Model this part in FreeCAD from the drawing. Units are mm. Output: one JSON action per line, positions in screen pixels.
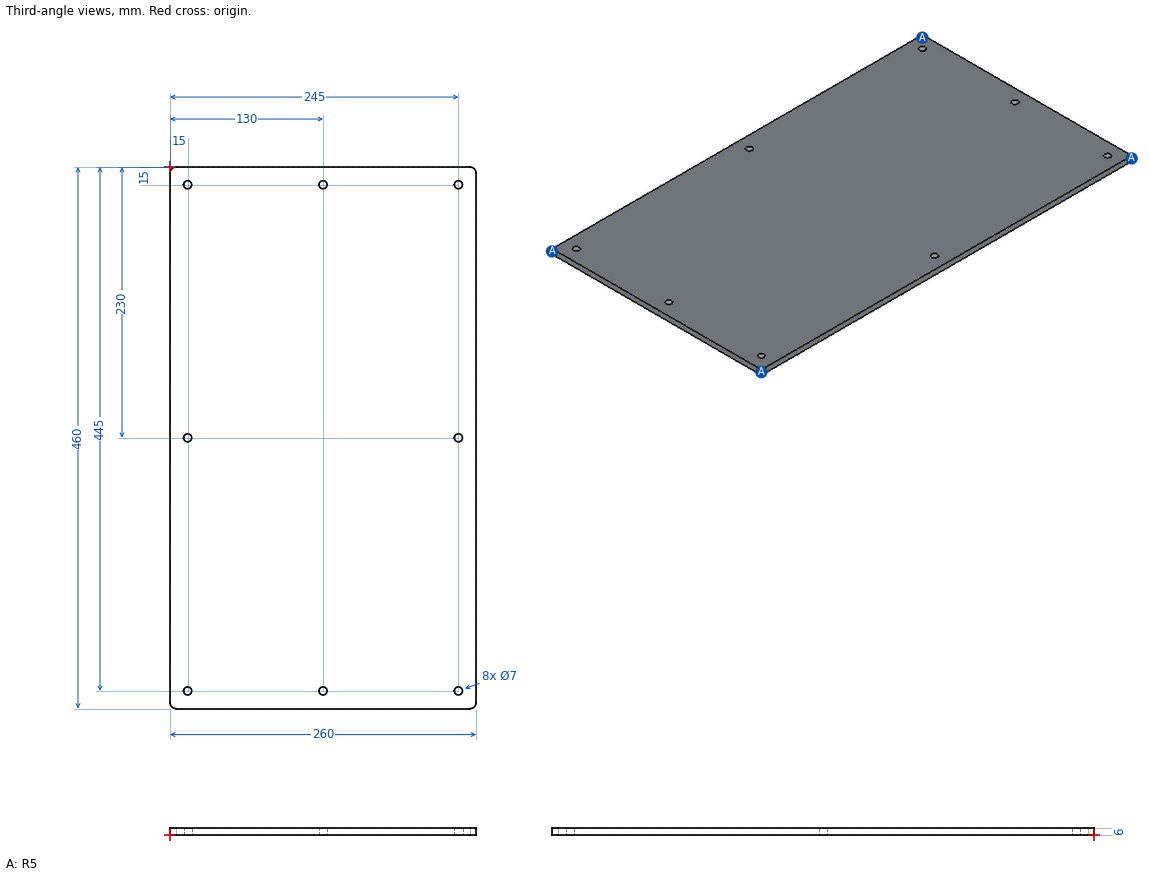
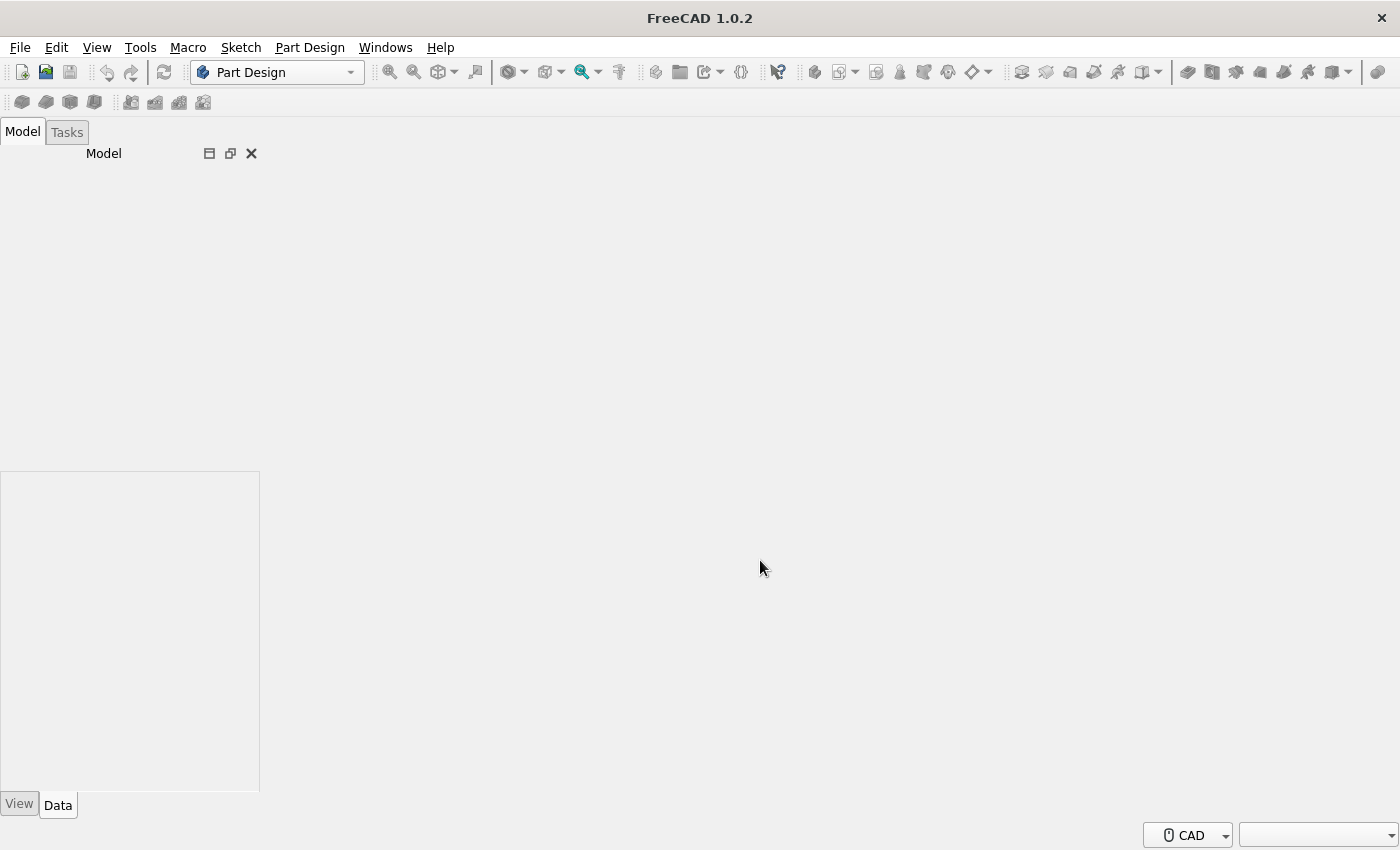
{"action": "key", "text": "ctrl+n"}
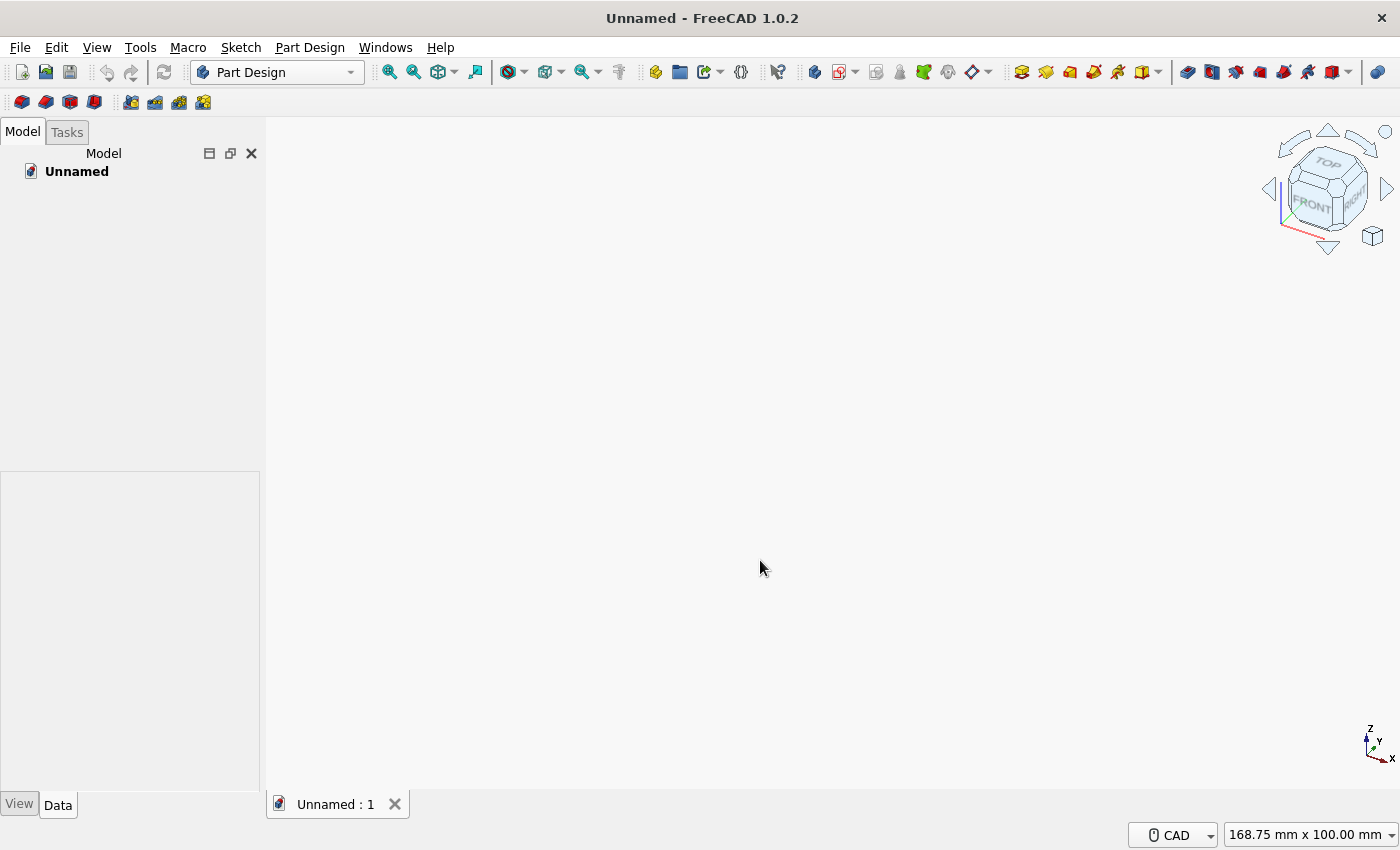
{"action": "left_click", "coordinate": [840, 72]}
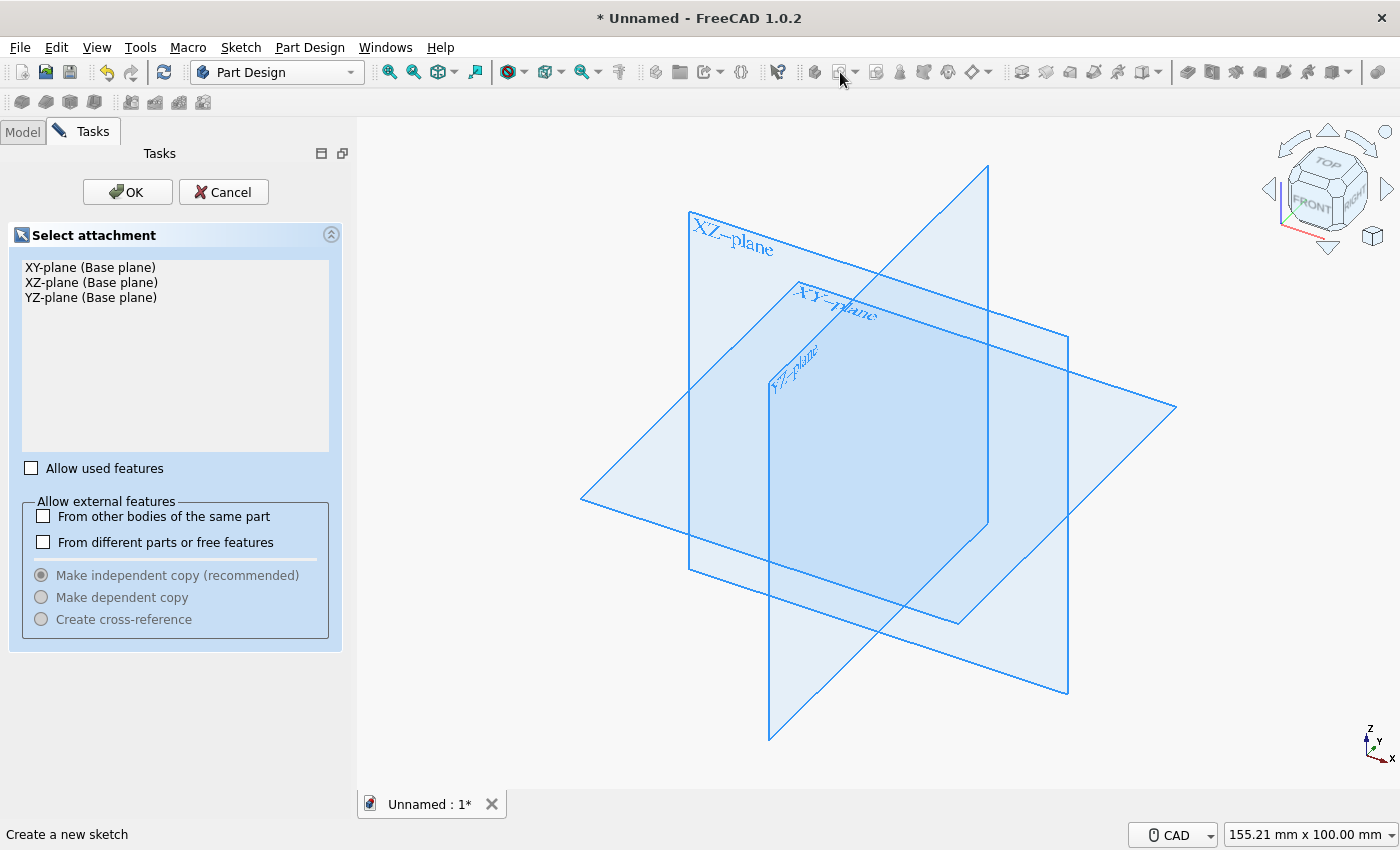
{"action": "left_click", "coordinate": [82, 268]}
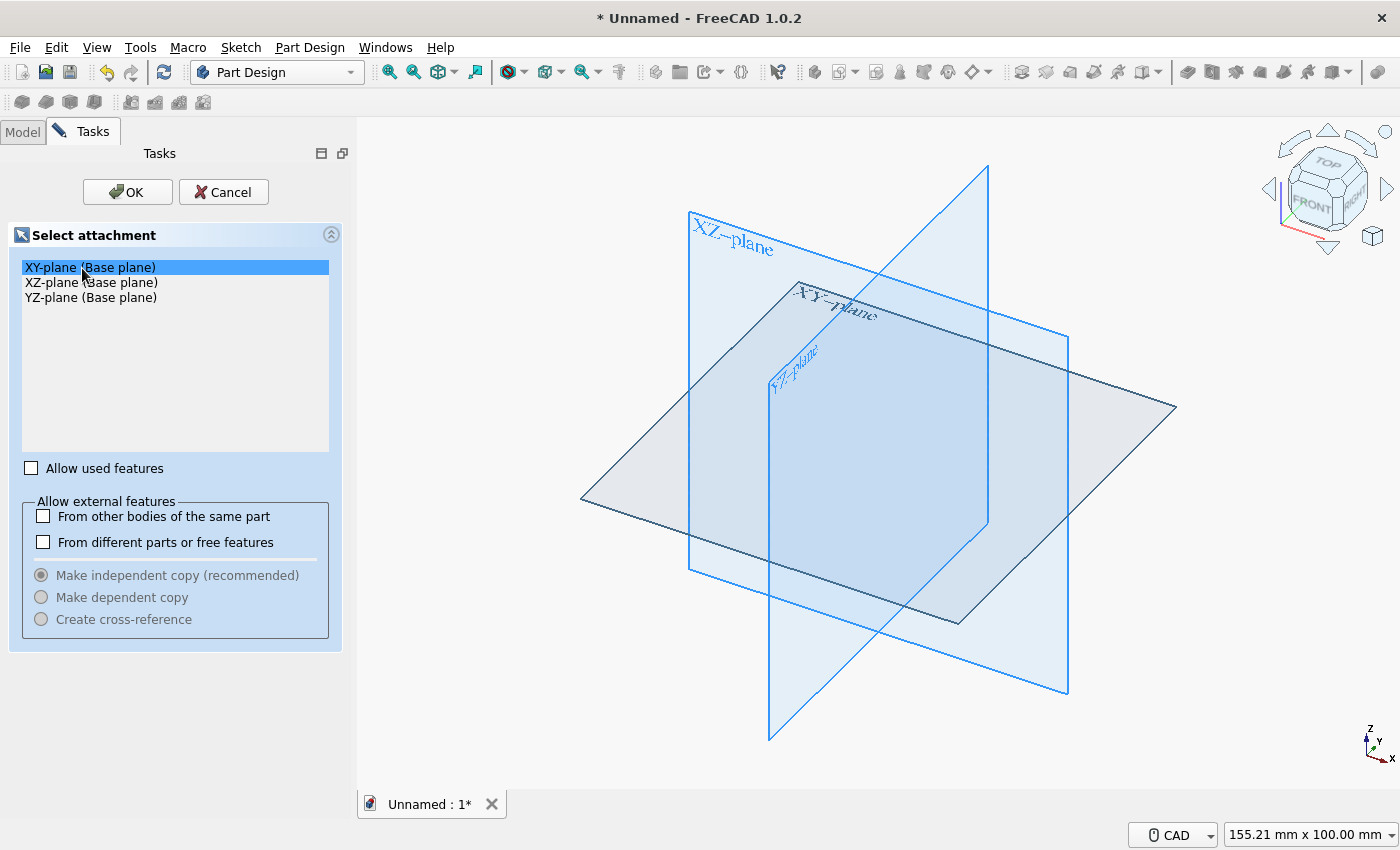
{"action": "left_click", "coordinate": [128, 192]}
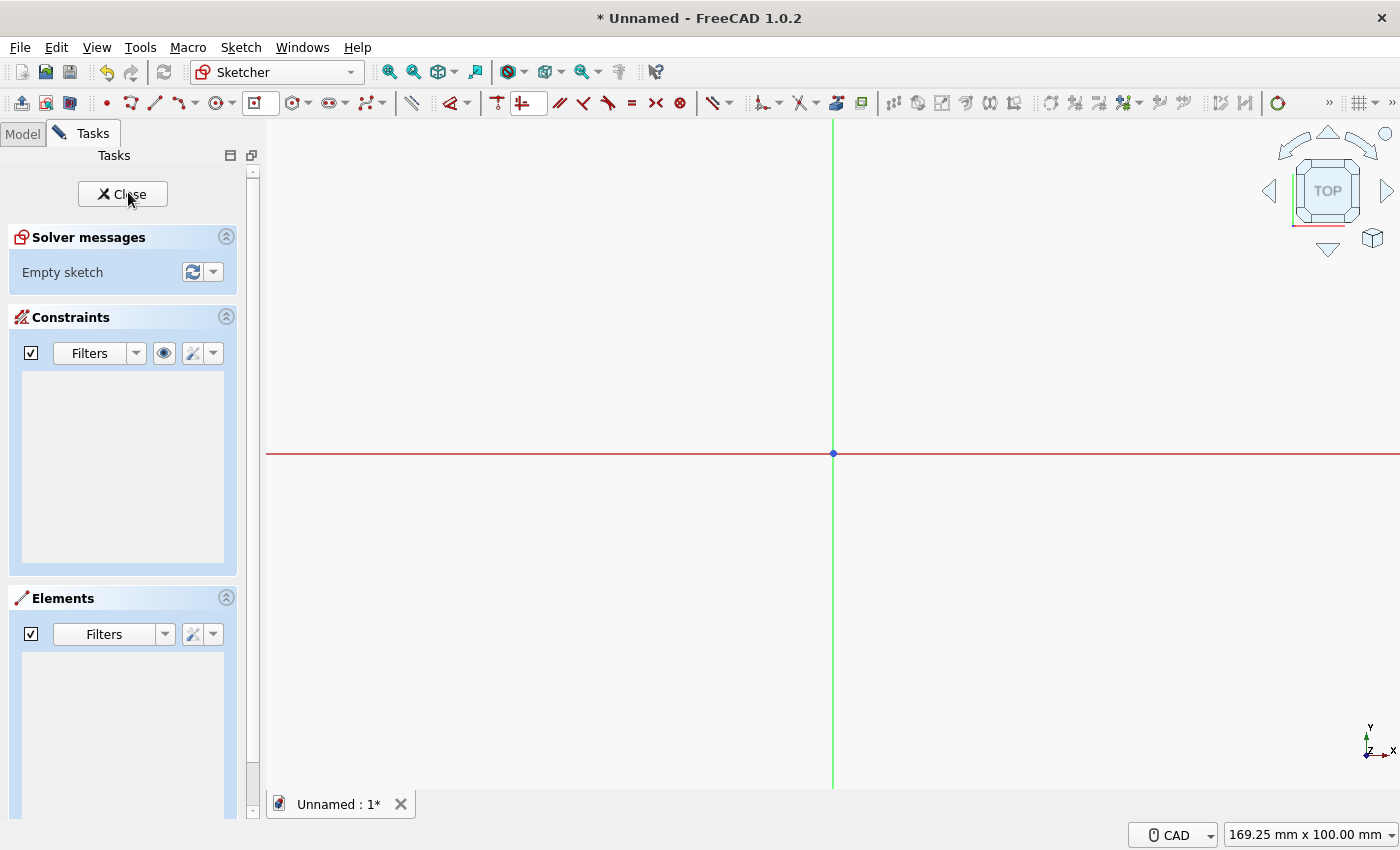
{"action": "scroll", "coordinate": [617, 213], "scroll_direction": "down", "scroll_amount": 10}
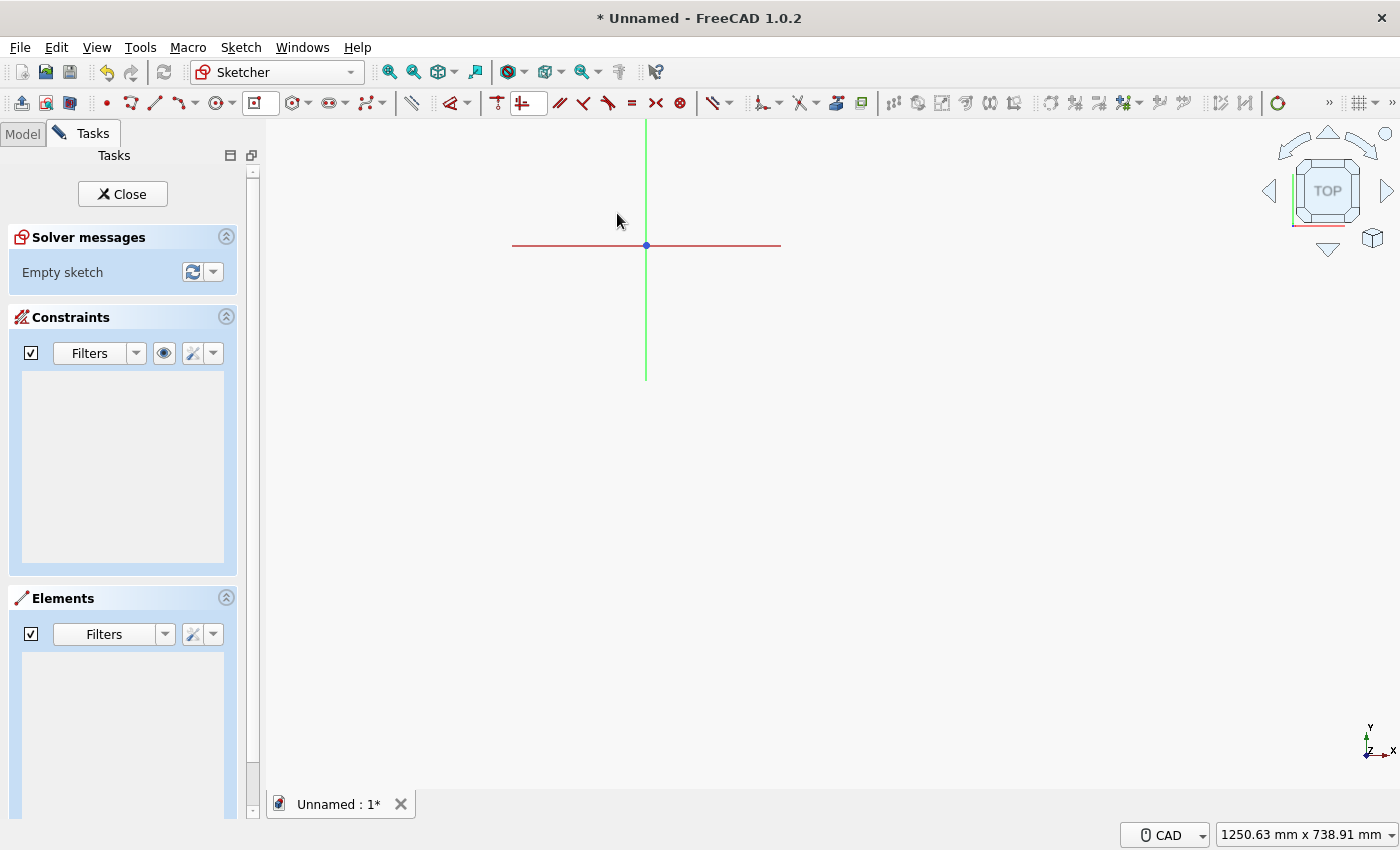
{"action": "key", "text": "g r"}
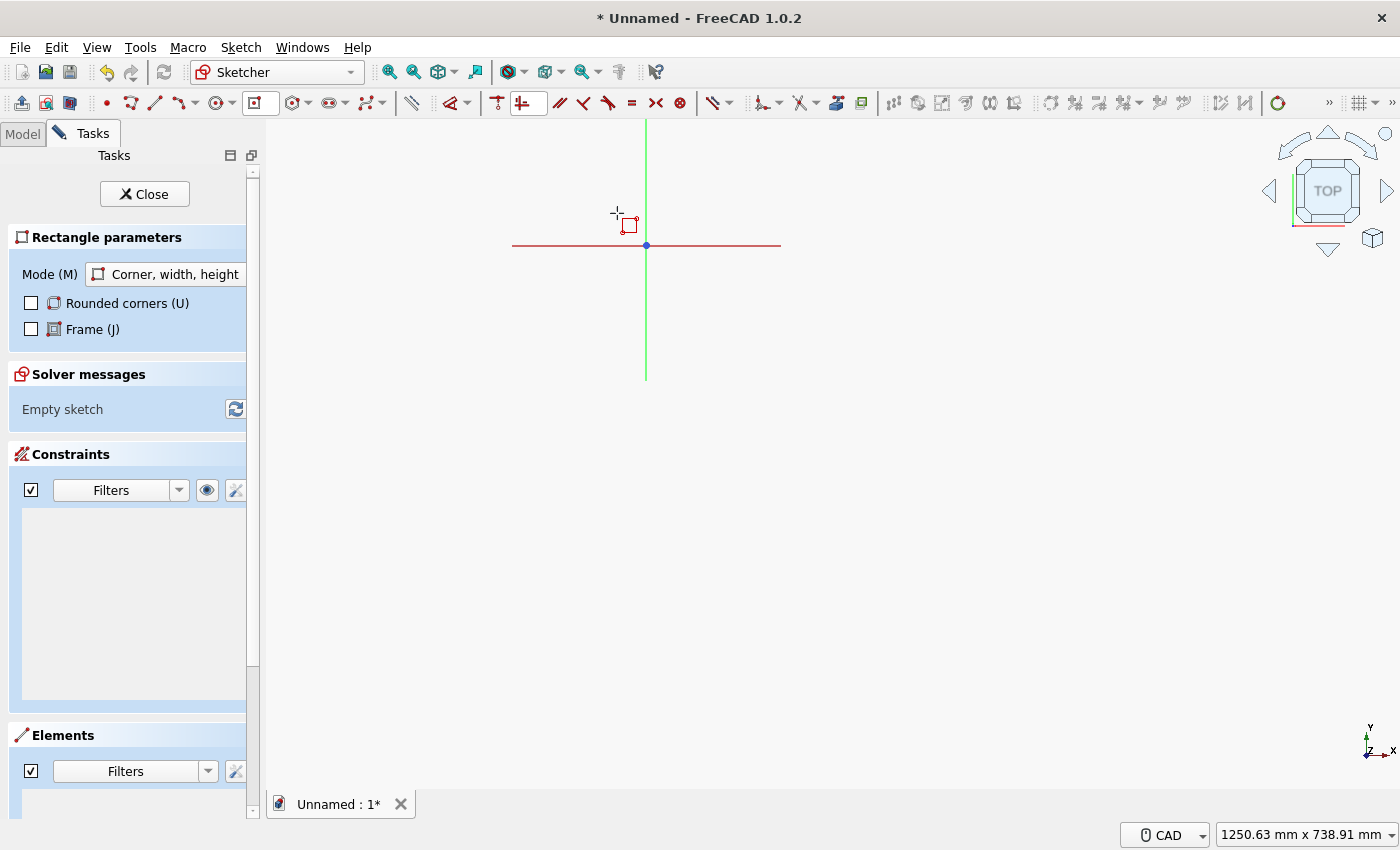
{"action": "left_click", "coordinate": [647, 246]}
{"action": "left_click", "coordinate": [882, 663]}
{"action": "key", "text": "Escape"}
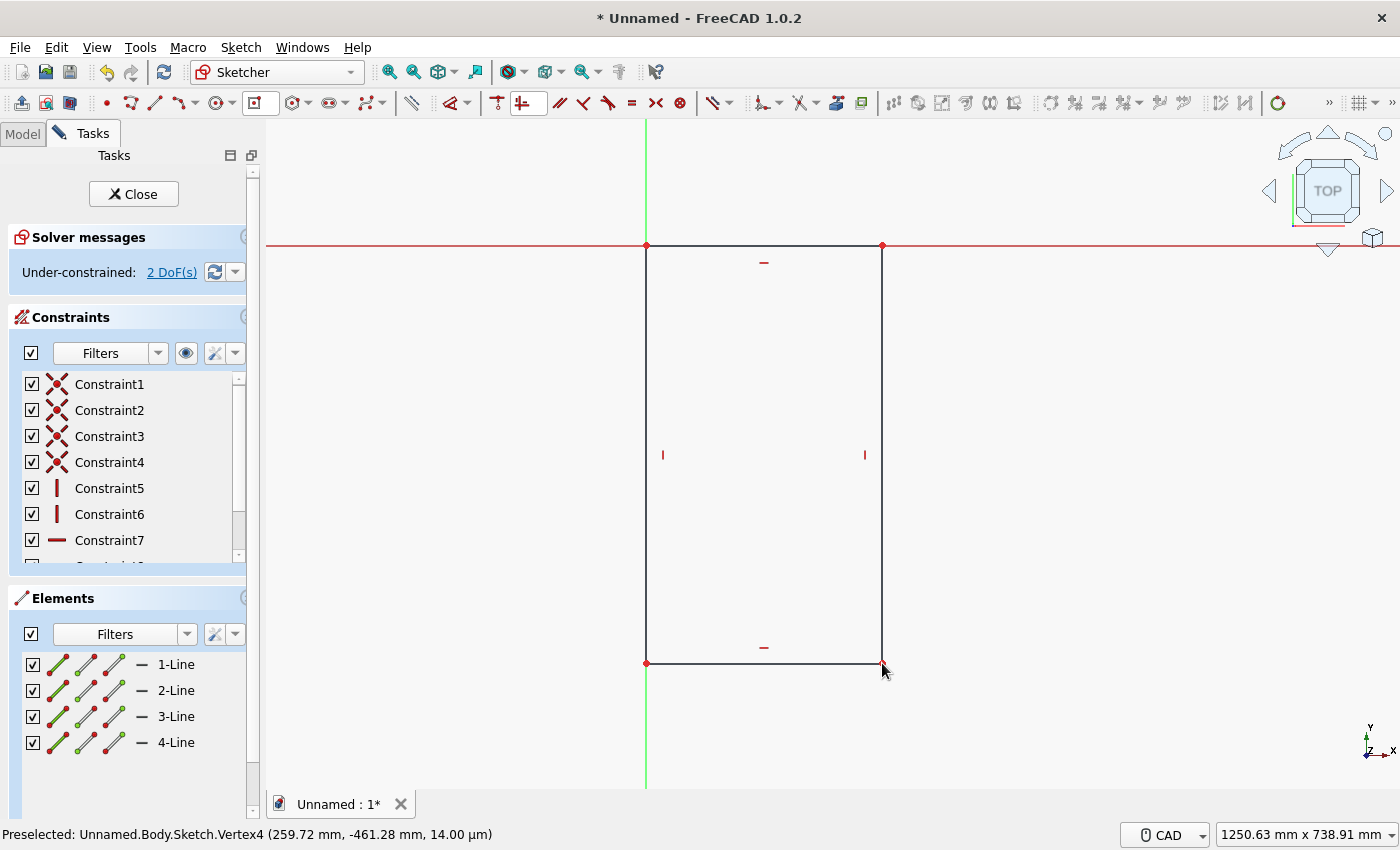
{"action": "left_click", "coordinate": [647, 371]}